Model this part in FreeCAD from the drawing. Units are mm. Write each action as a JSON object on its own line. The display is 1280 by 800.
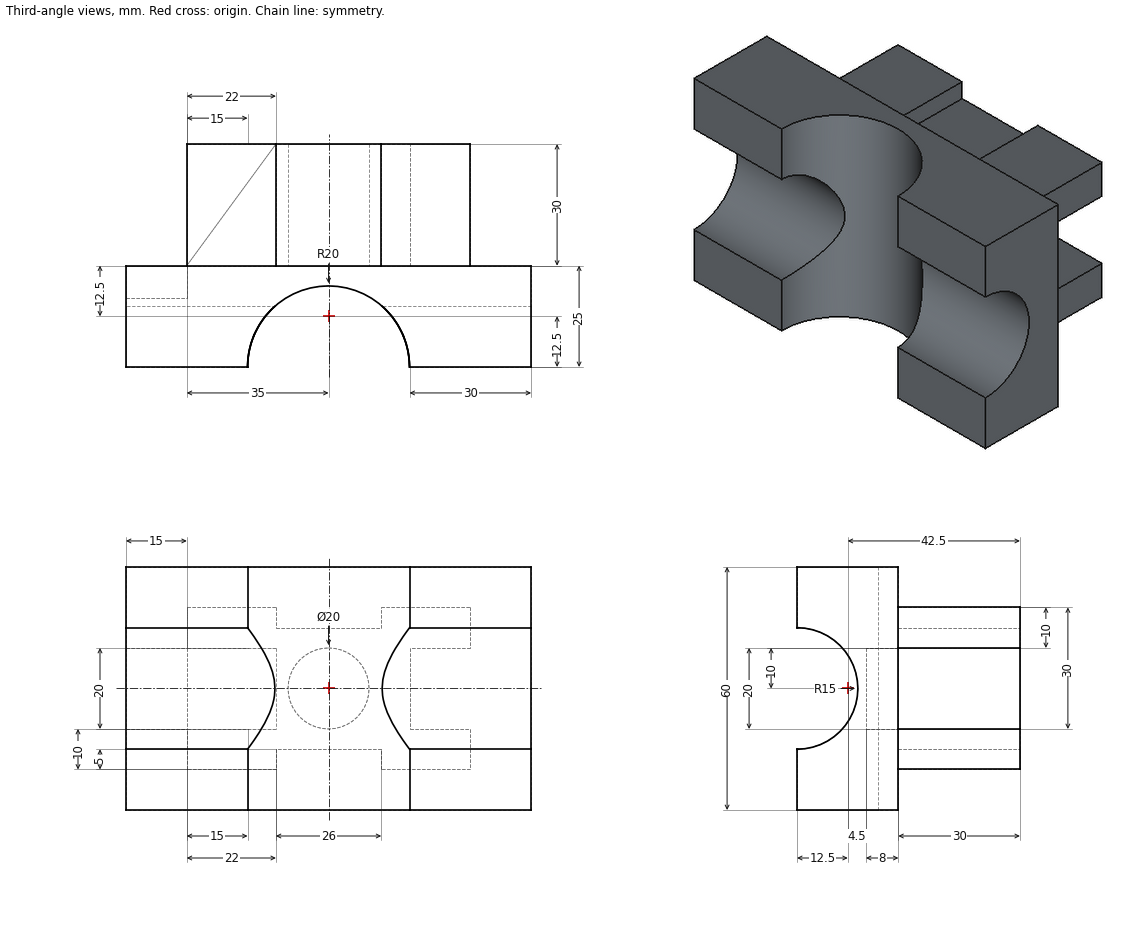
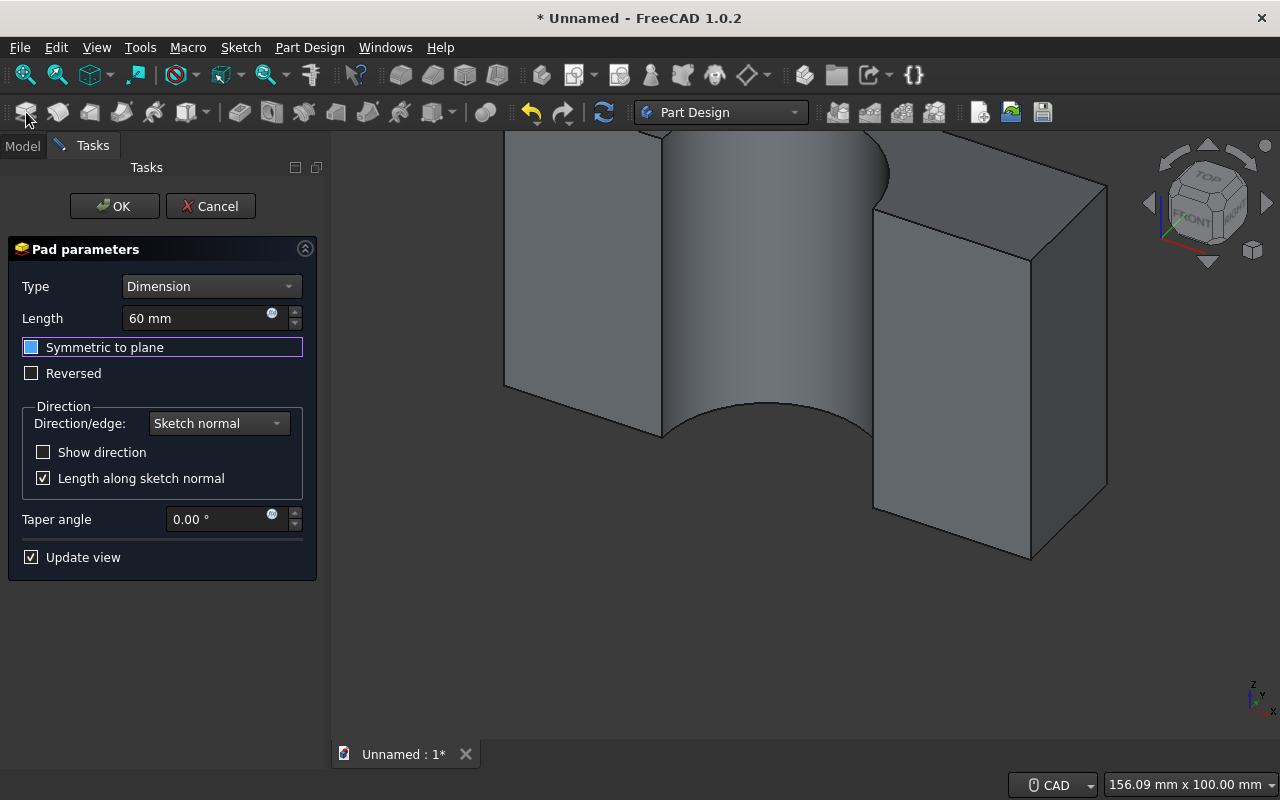
{"action": "left_click", "coordinate": [30, 347]}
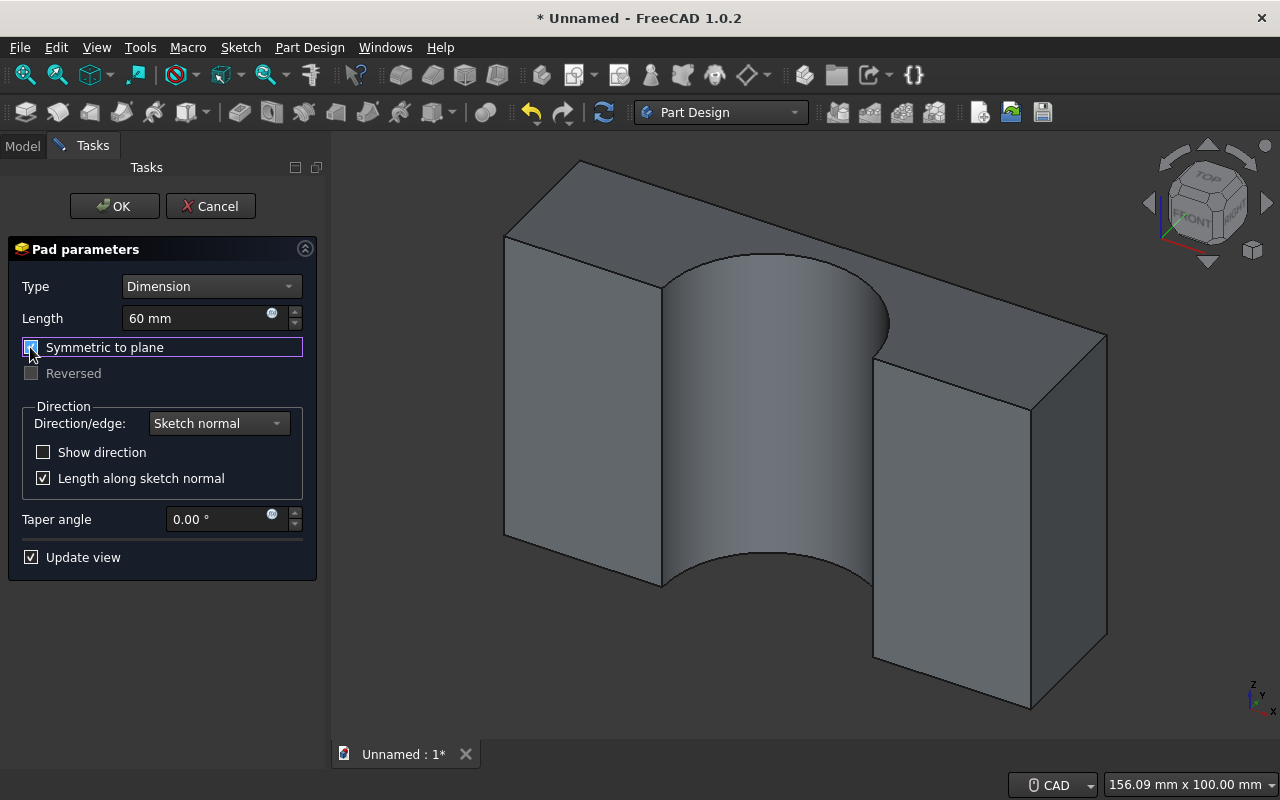
{"action": "left_click", "coordinate": [115, 206]}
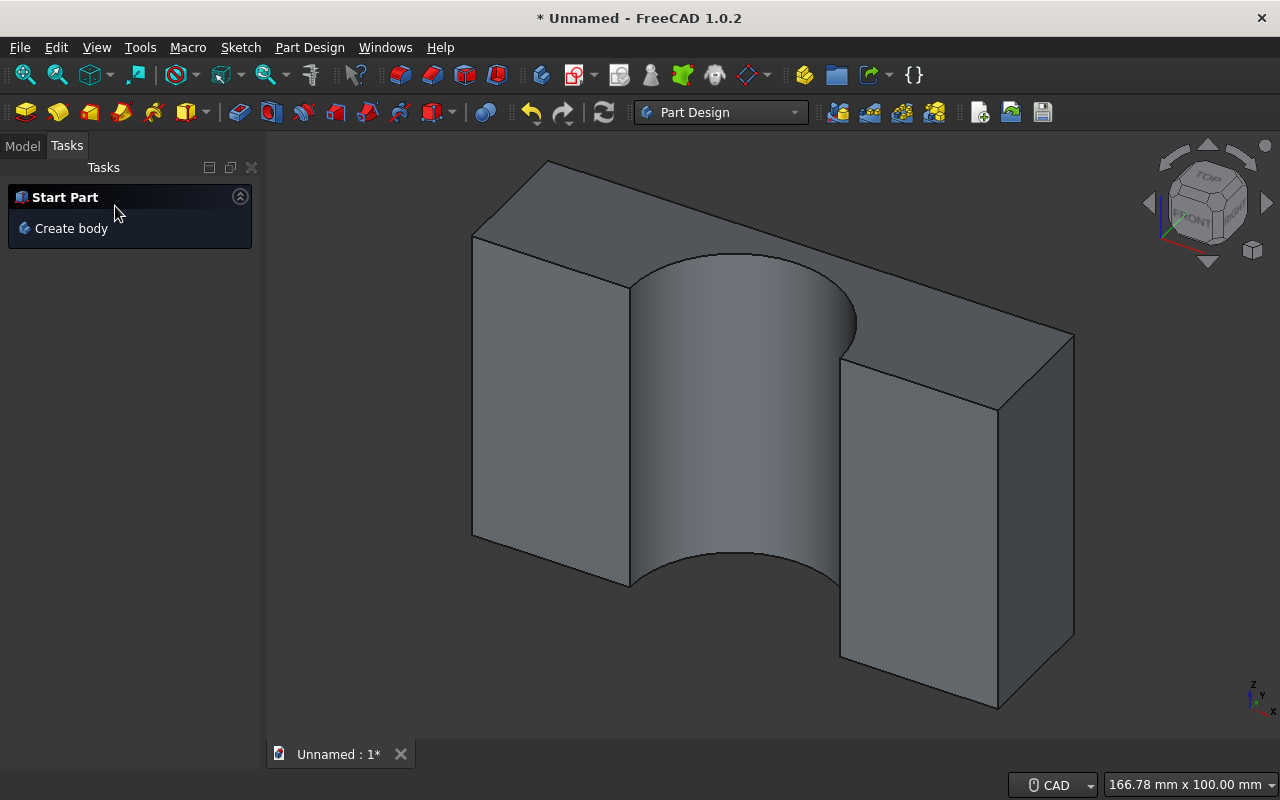
{"action": "key", "text": "6"}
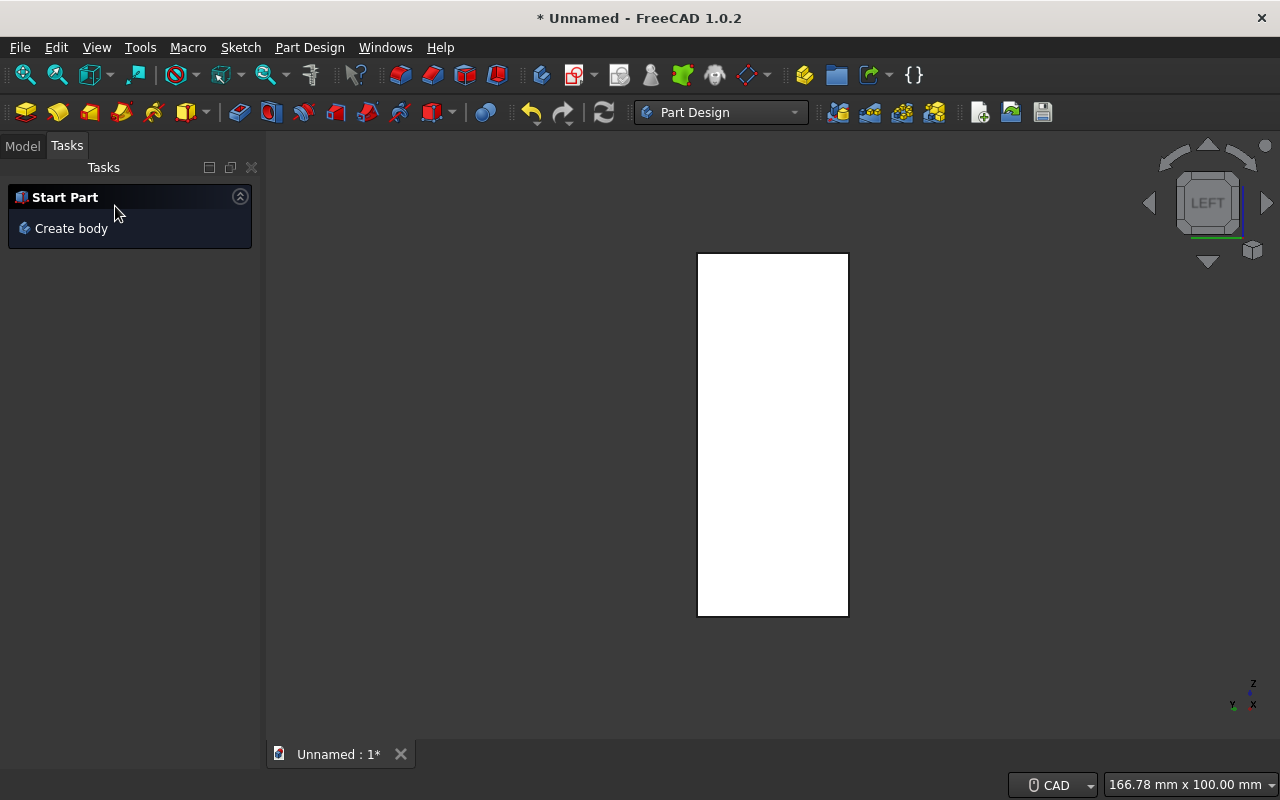
{"action": "left_click", "coordinate": [773, 330]}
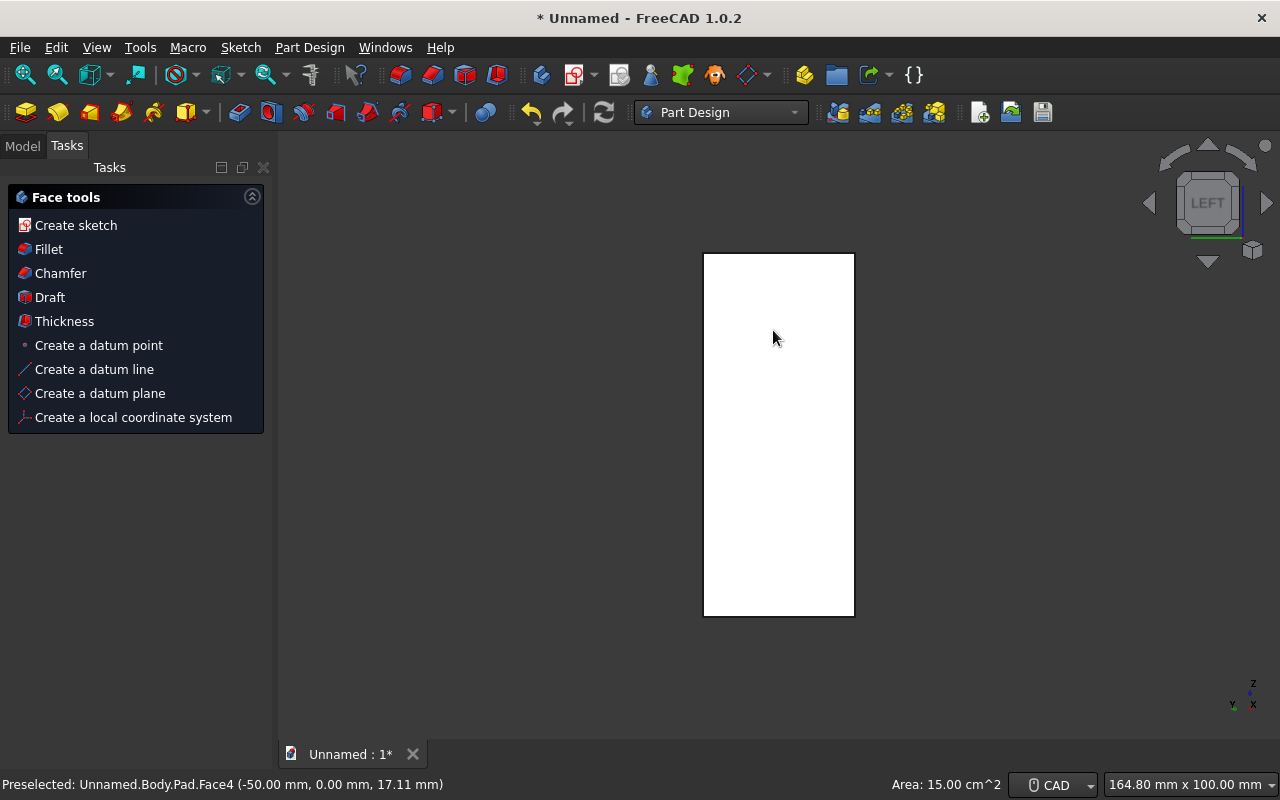
{"action": "left_click", "coordinate": [574, 76]}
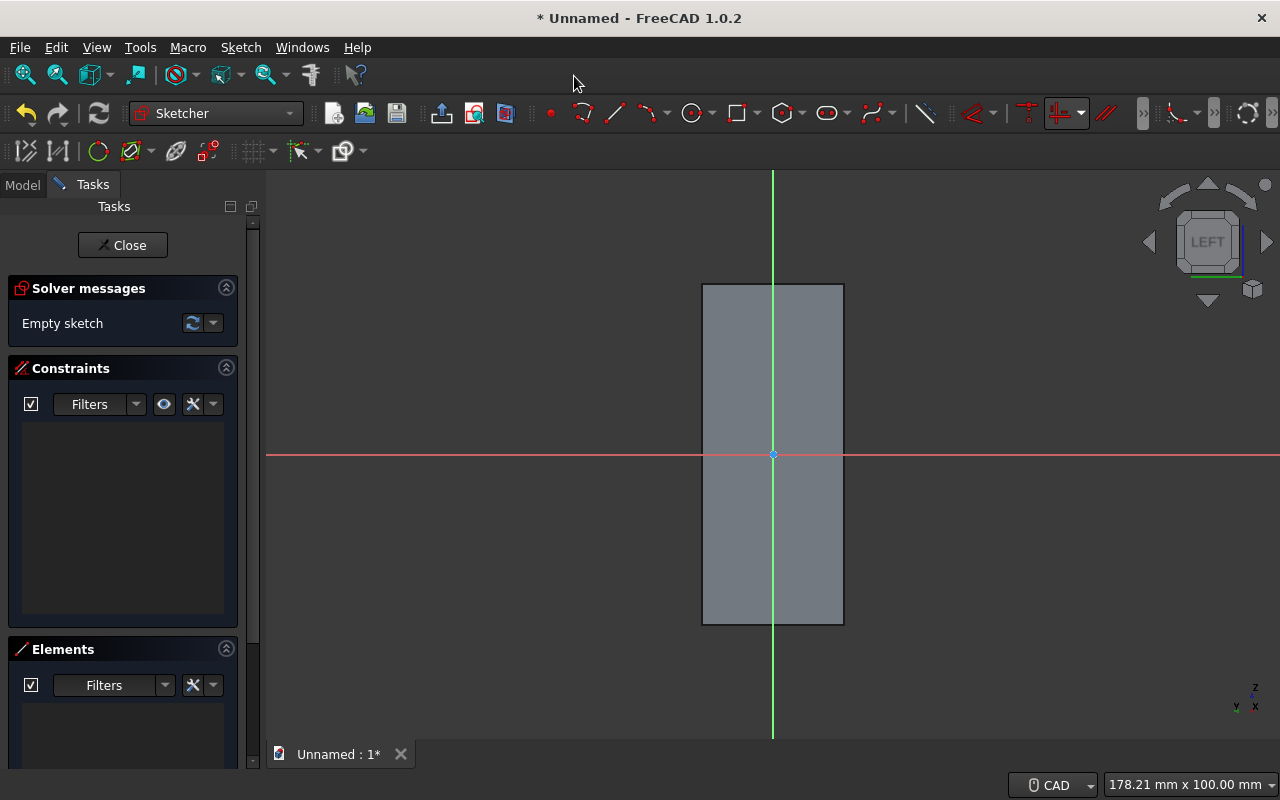
{"action": "scroll", "coordinate": [881, 455], "scroll_direction": "up", "scroll_amount": 4}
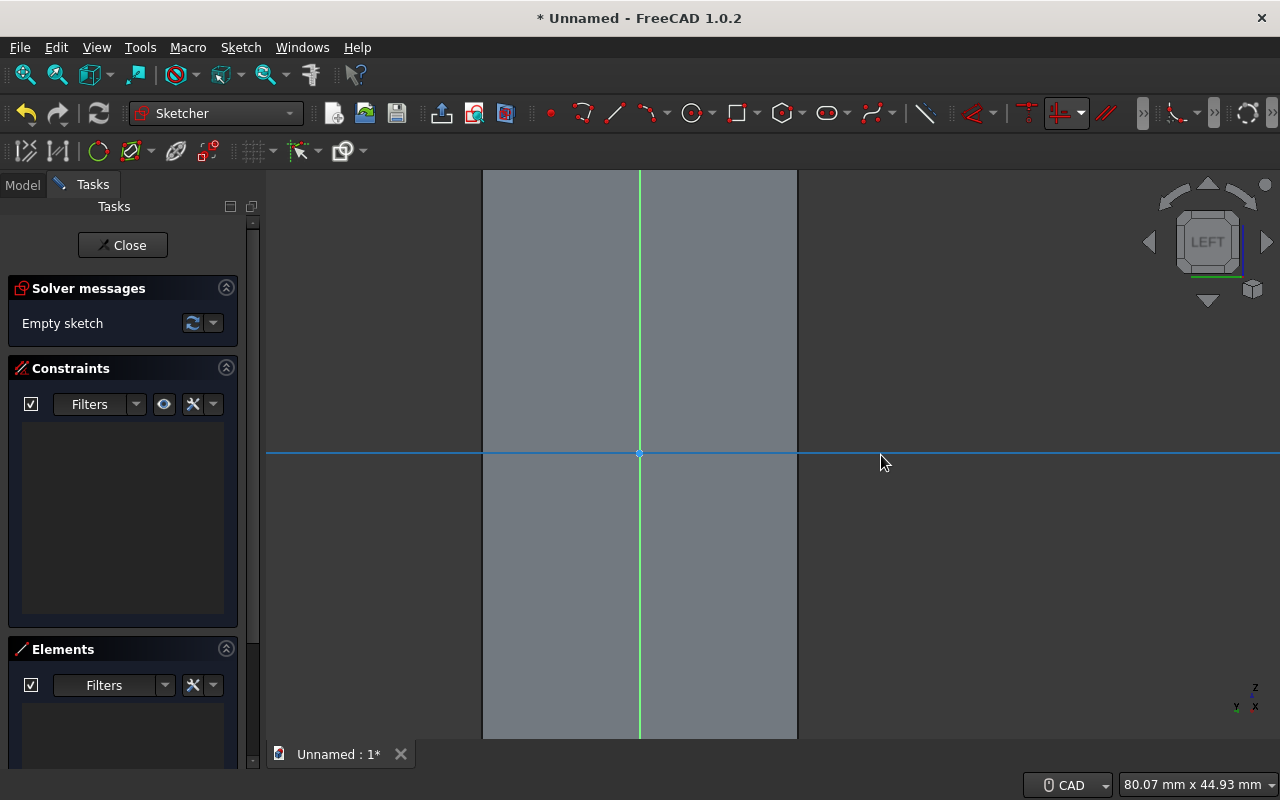
{"action": "left_click", "coordinate": [616, 114]}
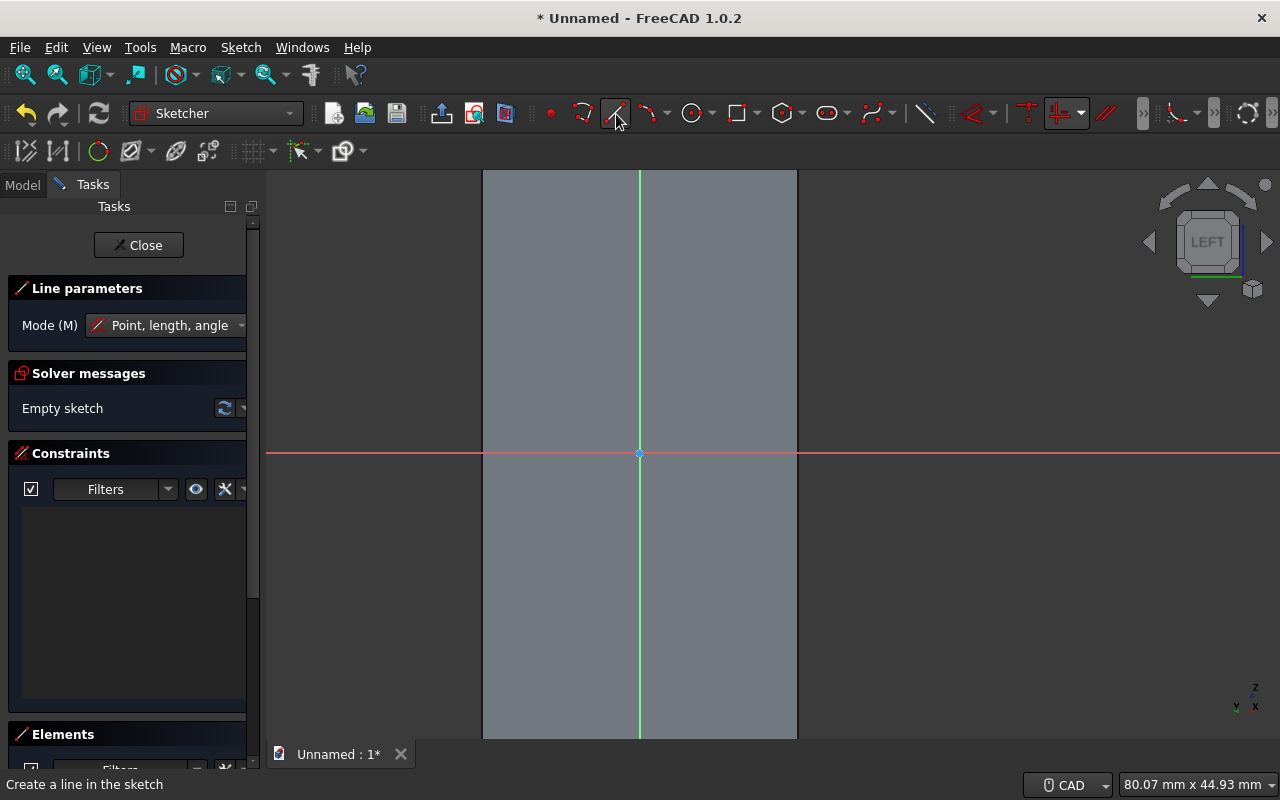
{"action": "left_click", "coordinate": [798, 643]}
{"action": "left_click", "coordinate": [798, 263]}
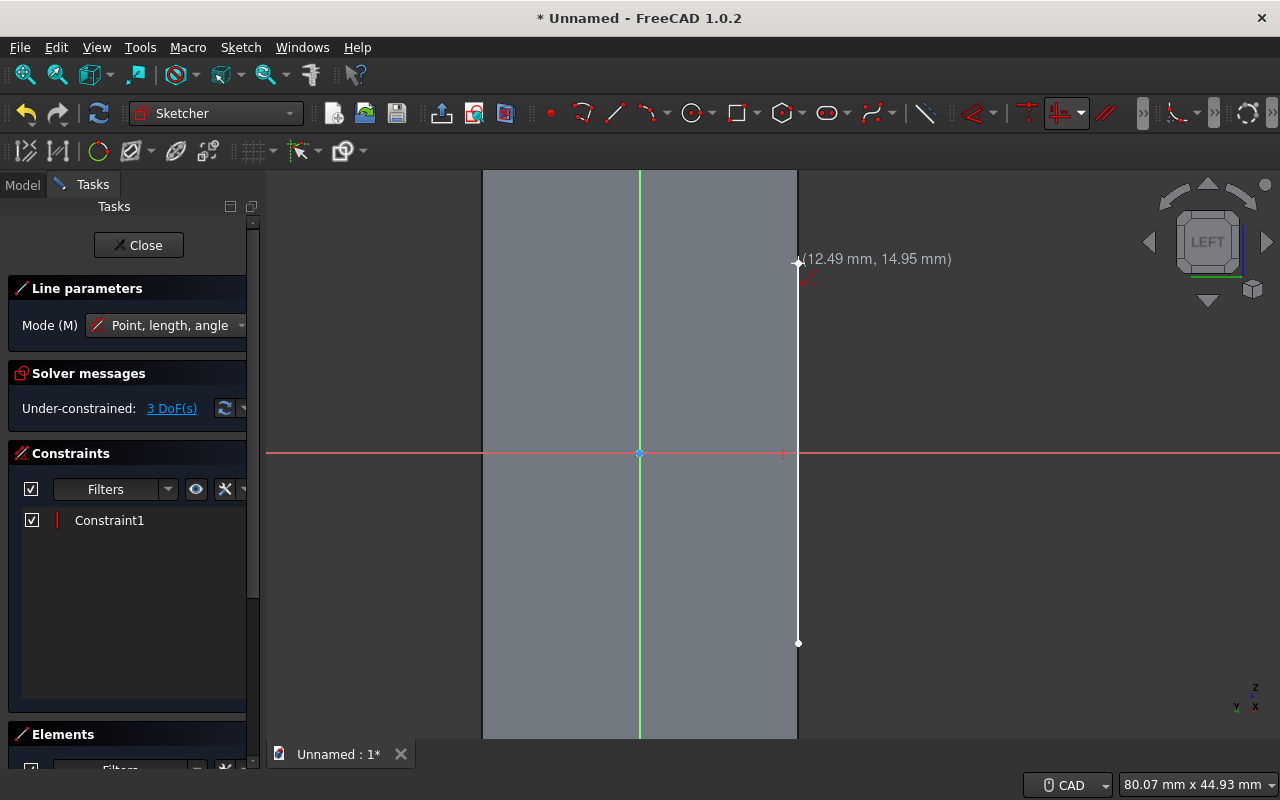
{"action": "left_click", "coordinate": [648, 114]}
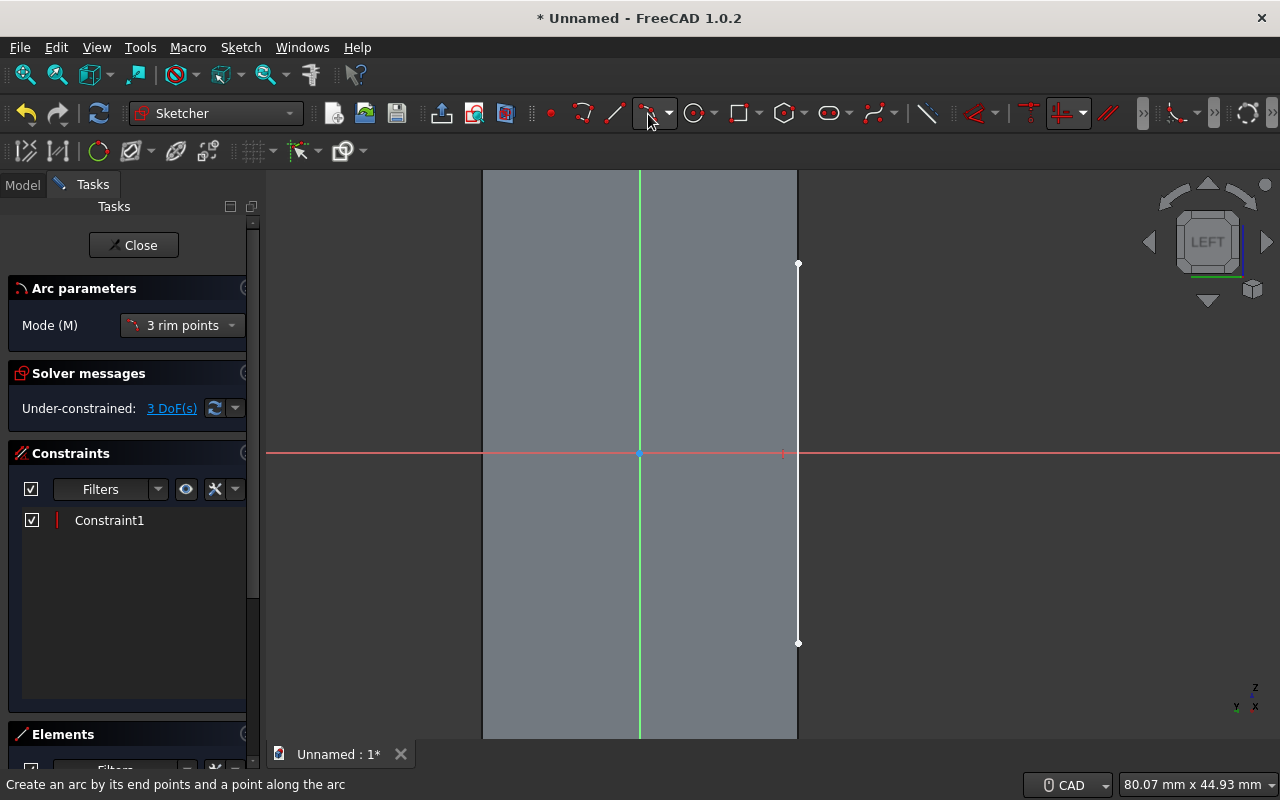
{"action": "left_click", "coordinate": [798, 264]}
{"action": "left_click", "coordinate": [798, 644]}
{"action": "left_click", "coordinate": [618, 395]}
{"action": "key", "text": "Escape"}